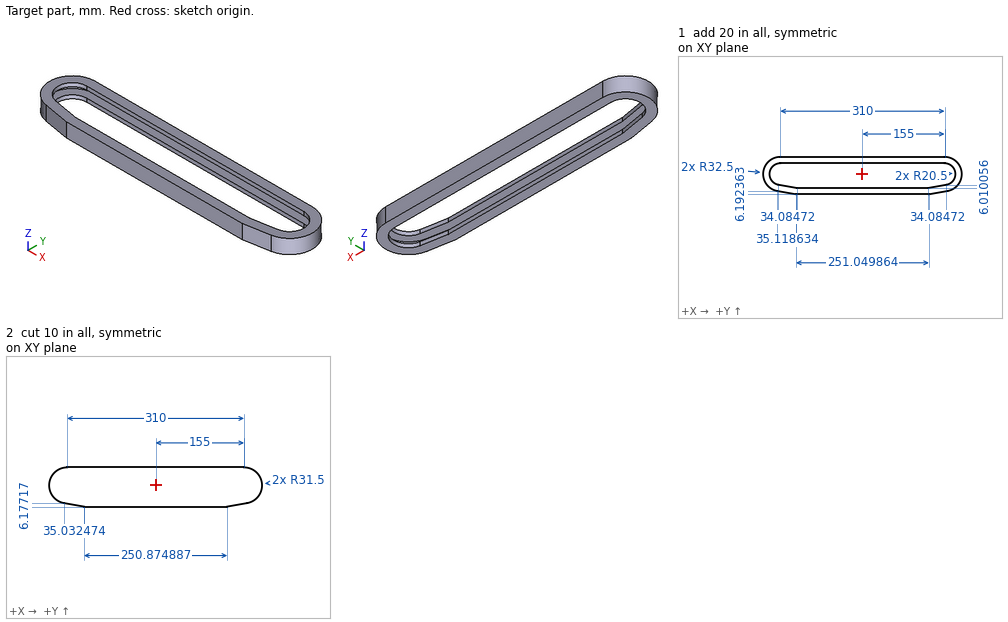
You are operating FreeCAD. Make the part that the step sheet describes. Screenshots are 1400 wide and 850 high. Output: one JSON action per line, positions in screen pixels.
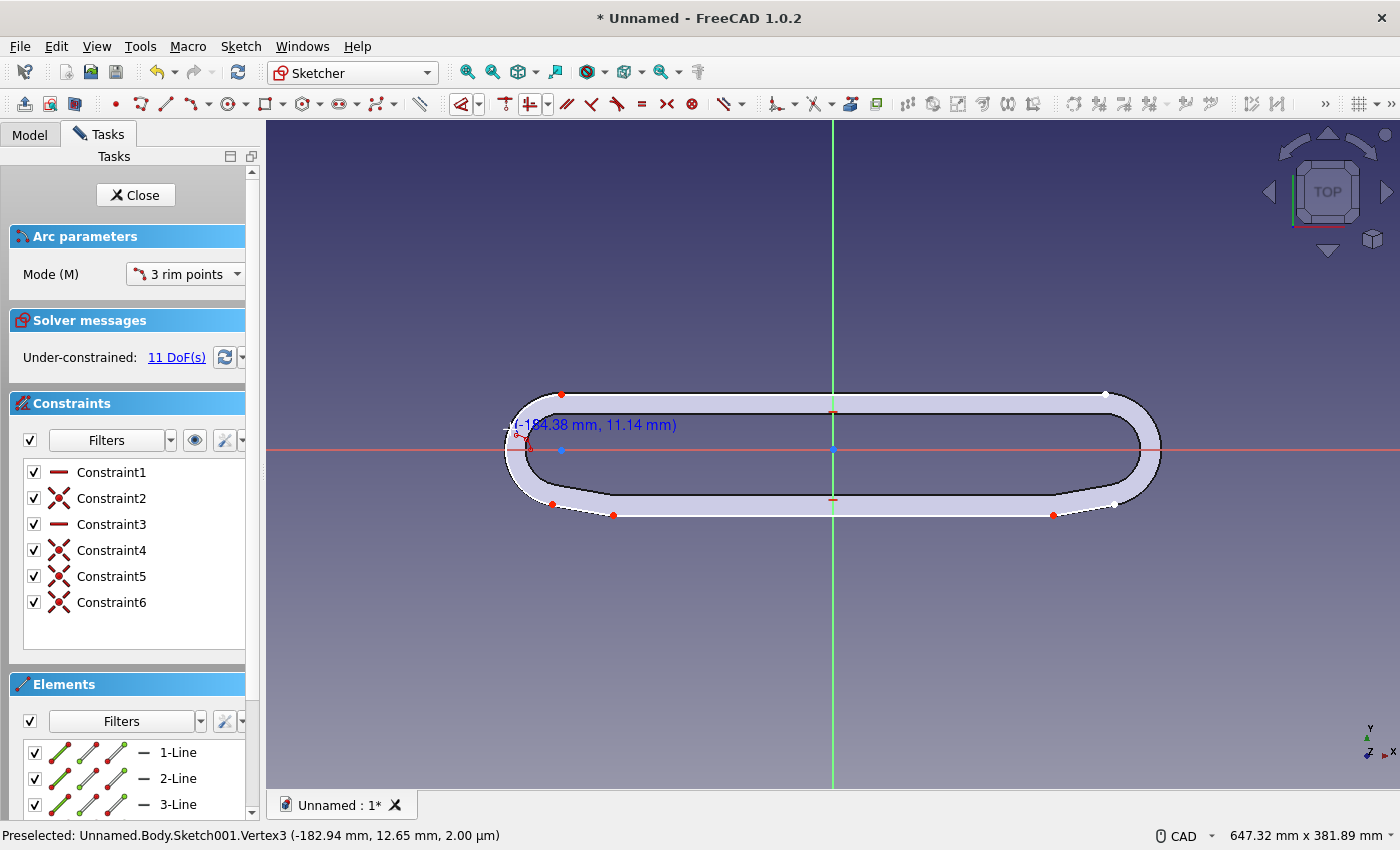
{"action": "left_click", "coordinate": [1114, 505]}
{"action": "left_click", "coordinate": [1105, 395]}
{"action": "left_click", "coordinate": [1156, 429]}
{"action": "key", "text": "Escape"}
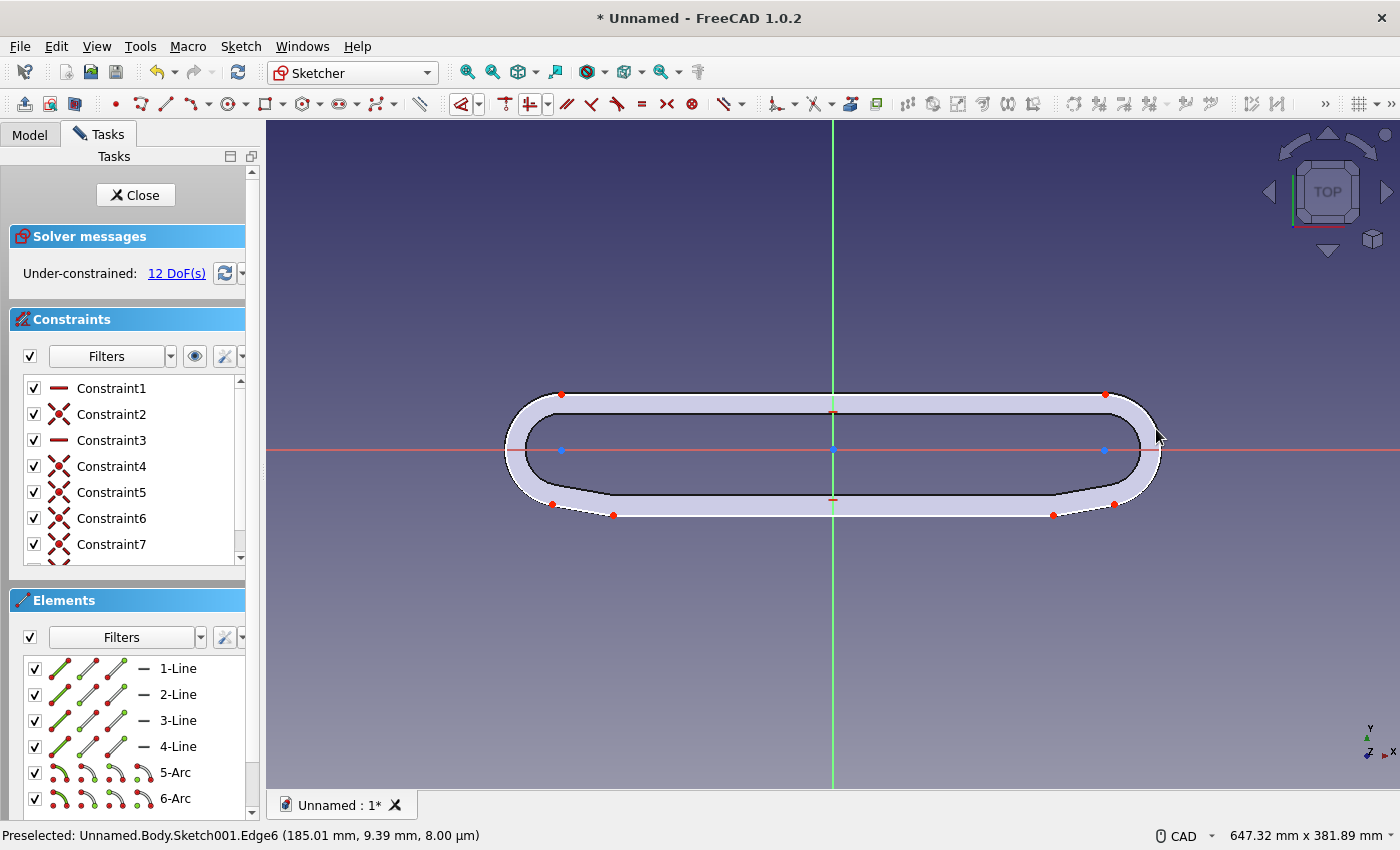
{"action": "left_click", "coordinate": [942, 395]}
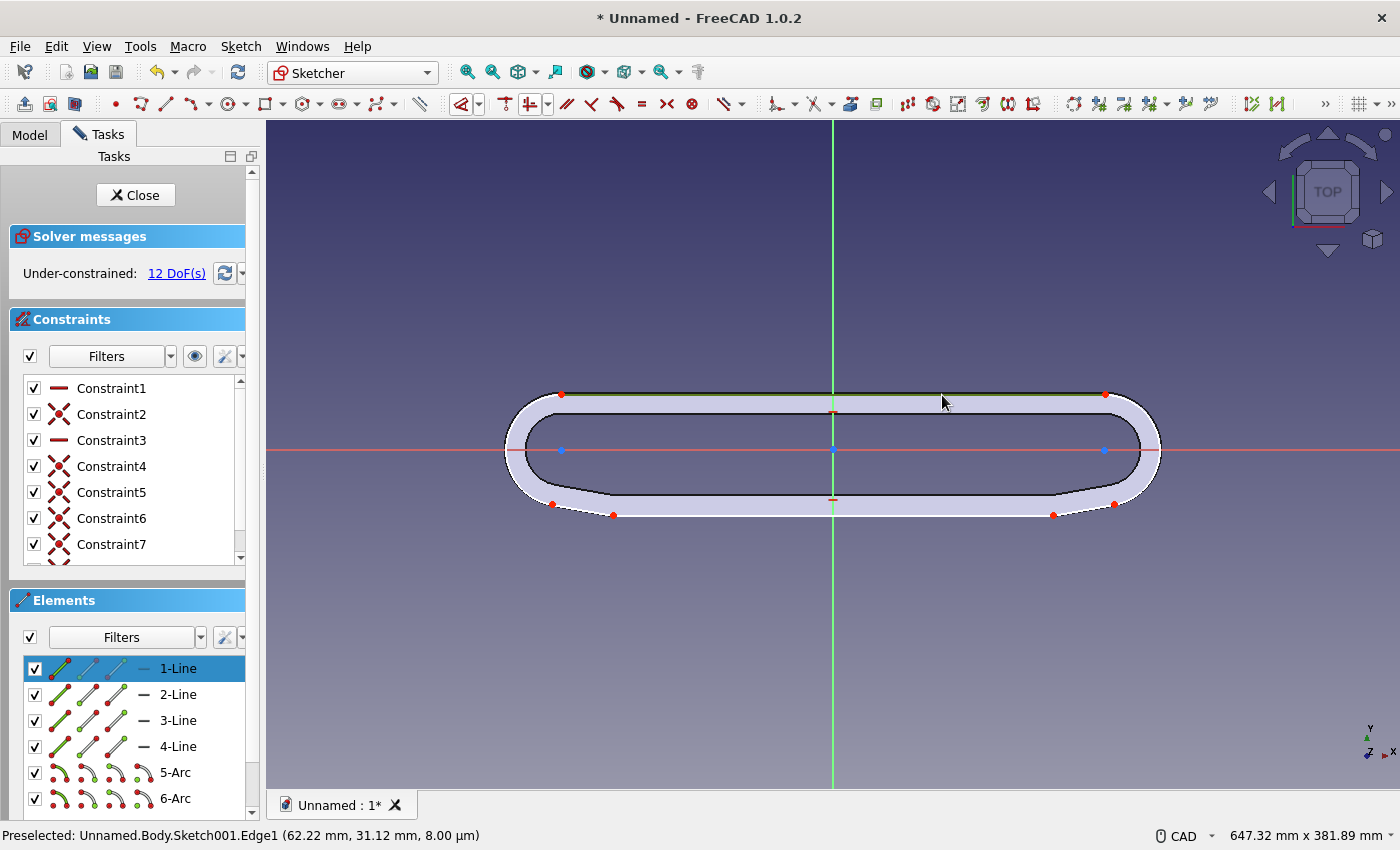
{"action": "left_click", "coordinate": [518, 416]}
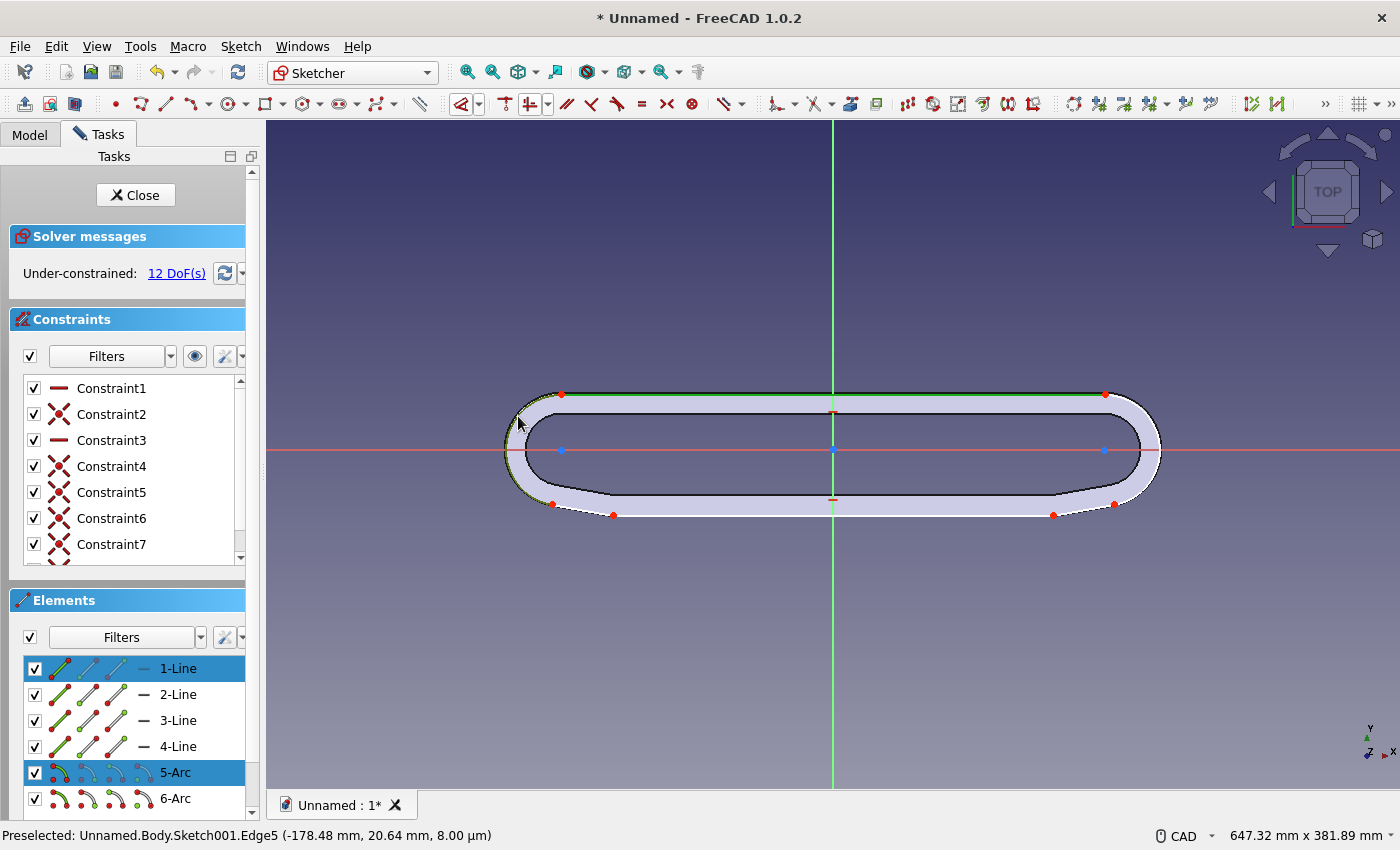
{"action": "key", "text": "t"}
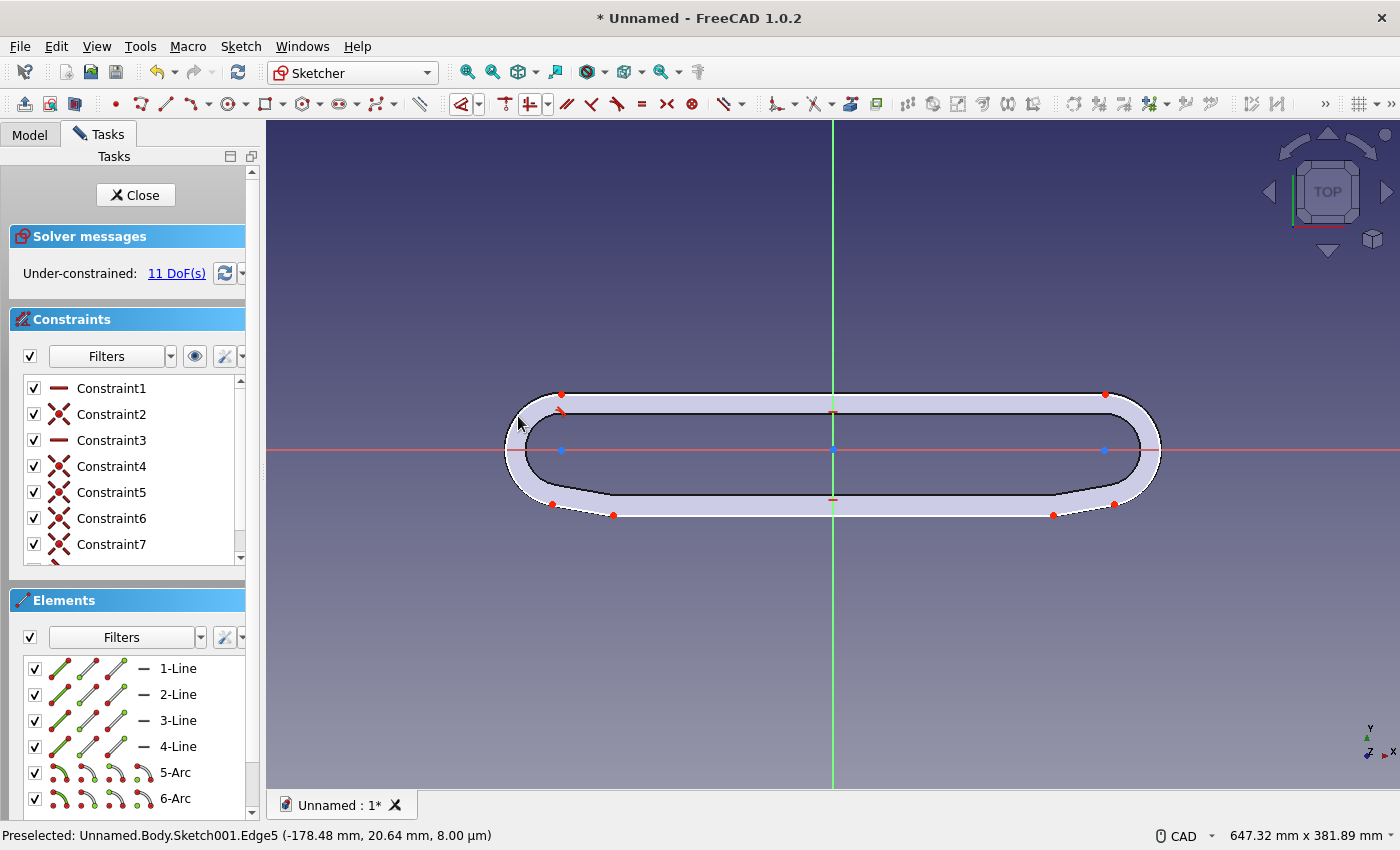
{"action": "left_click", "coordinate": [942, 395]}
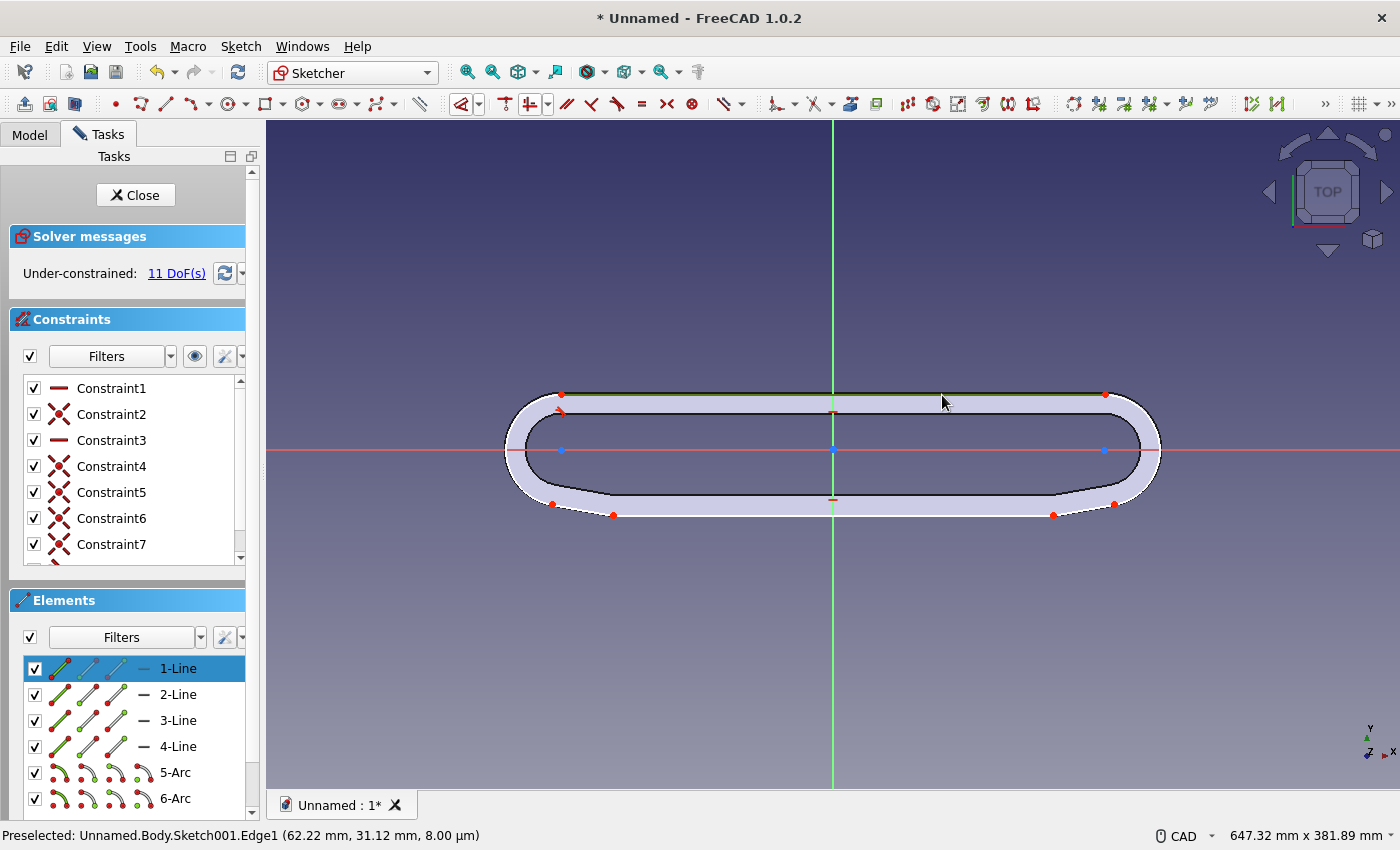
{"action": "left_click", "coordinate": [1153, 477]}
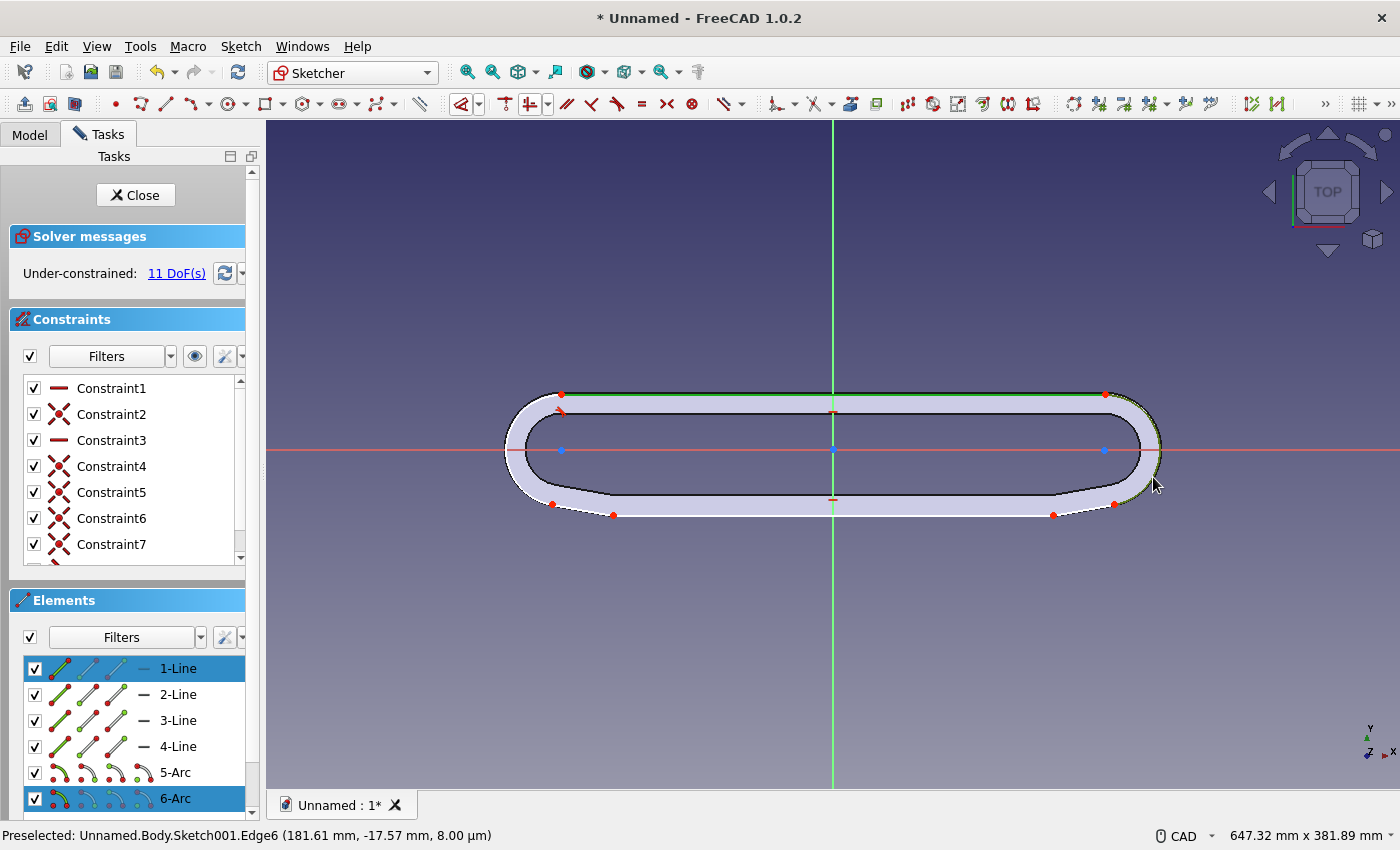
{"action": "left_click", "coordinate": [617, 104]}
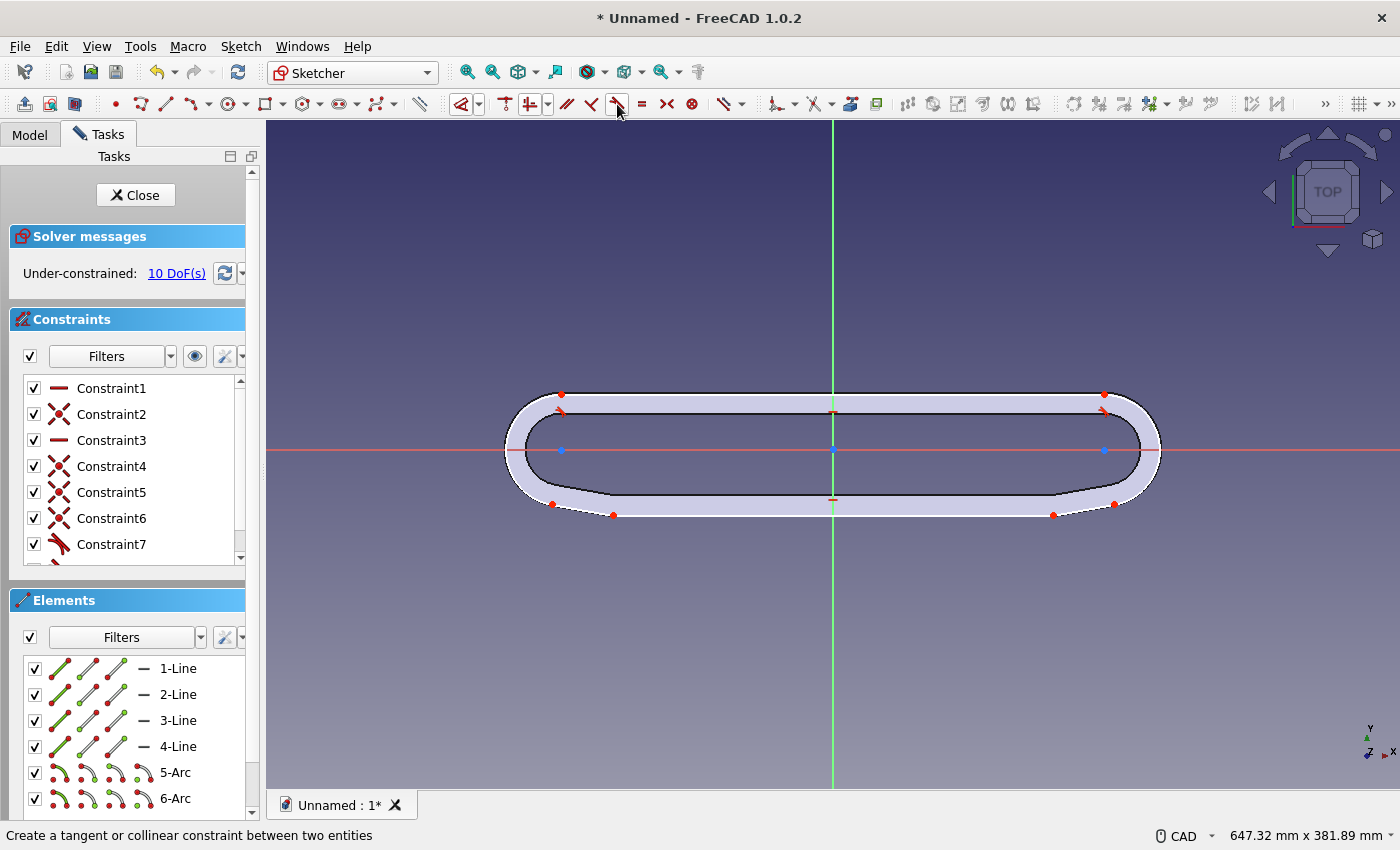
{"action": "left_click", "coordinate": [570, 508]}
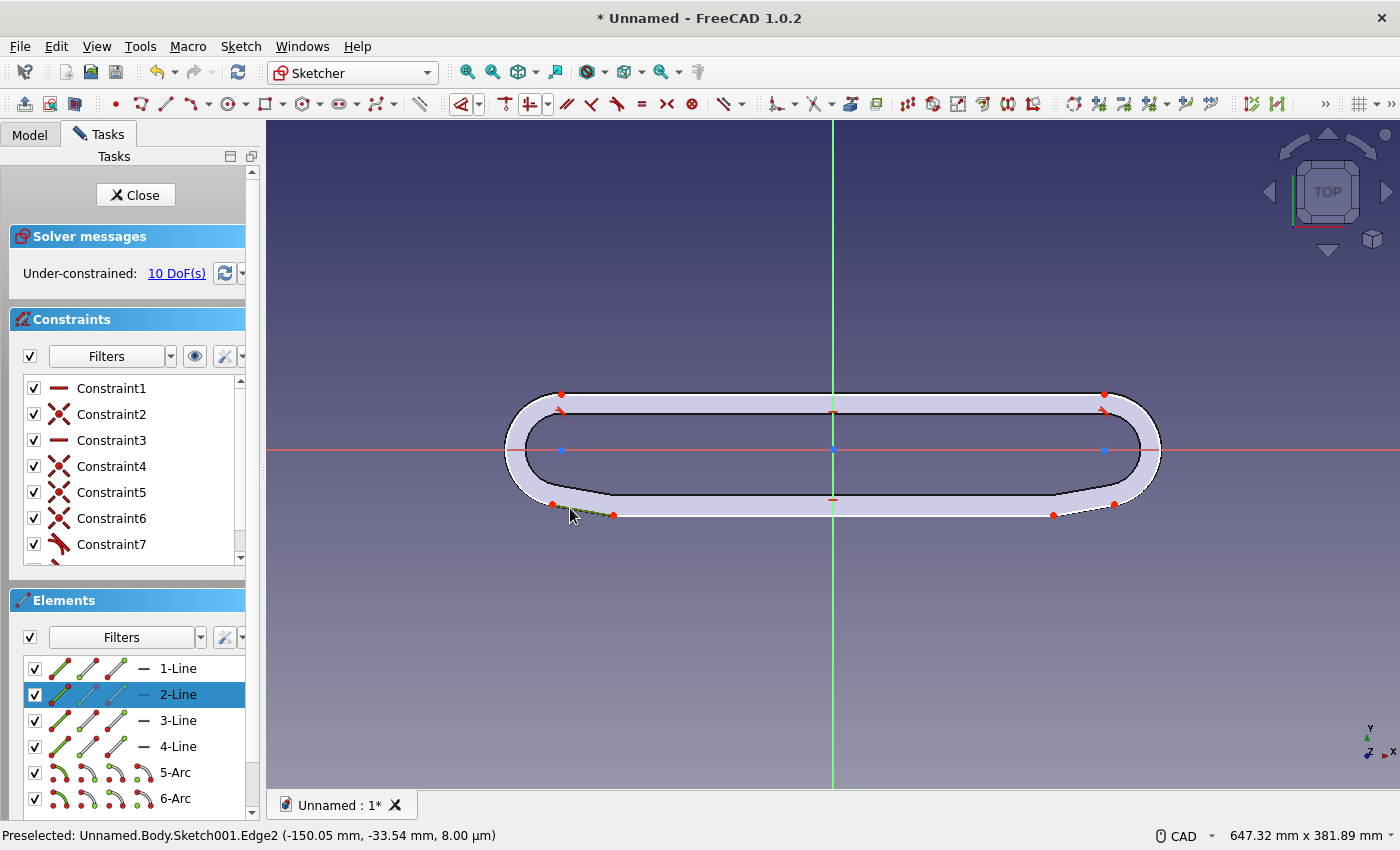
{"action": "left_click", "coordinate": [518, 416]}